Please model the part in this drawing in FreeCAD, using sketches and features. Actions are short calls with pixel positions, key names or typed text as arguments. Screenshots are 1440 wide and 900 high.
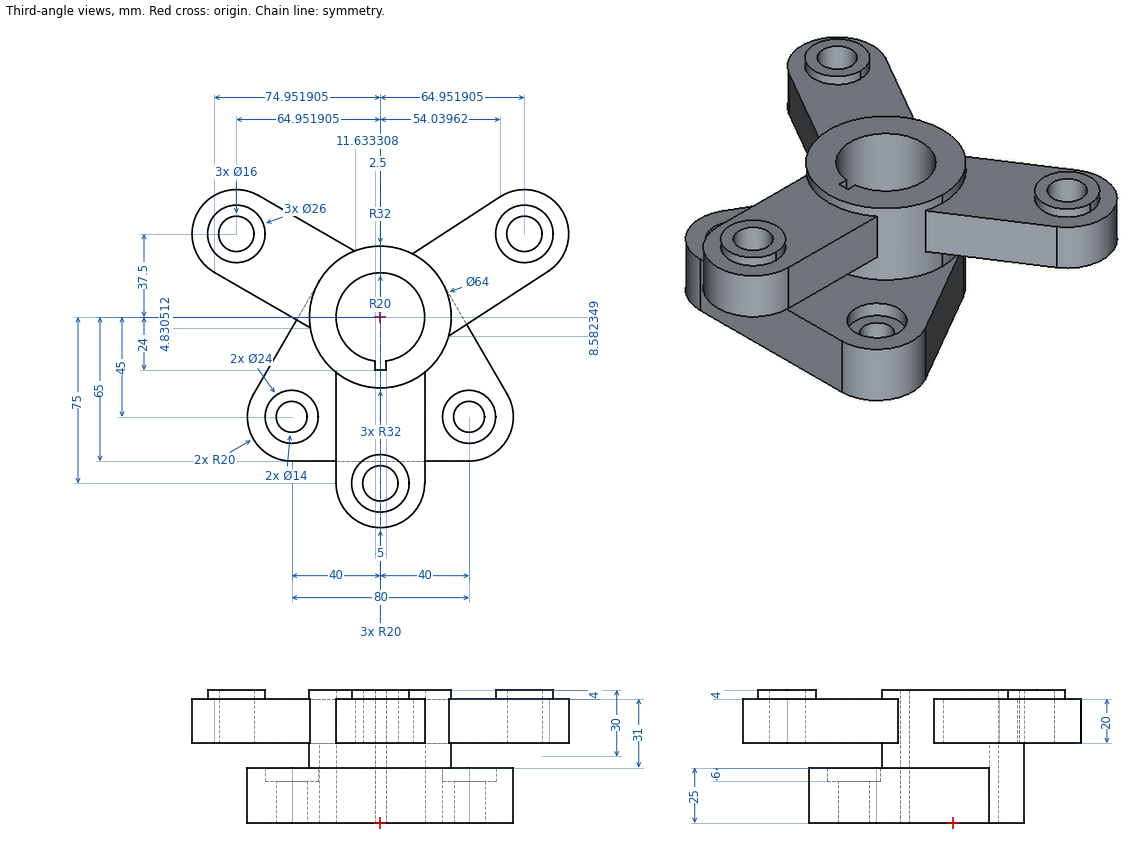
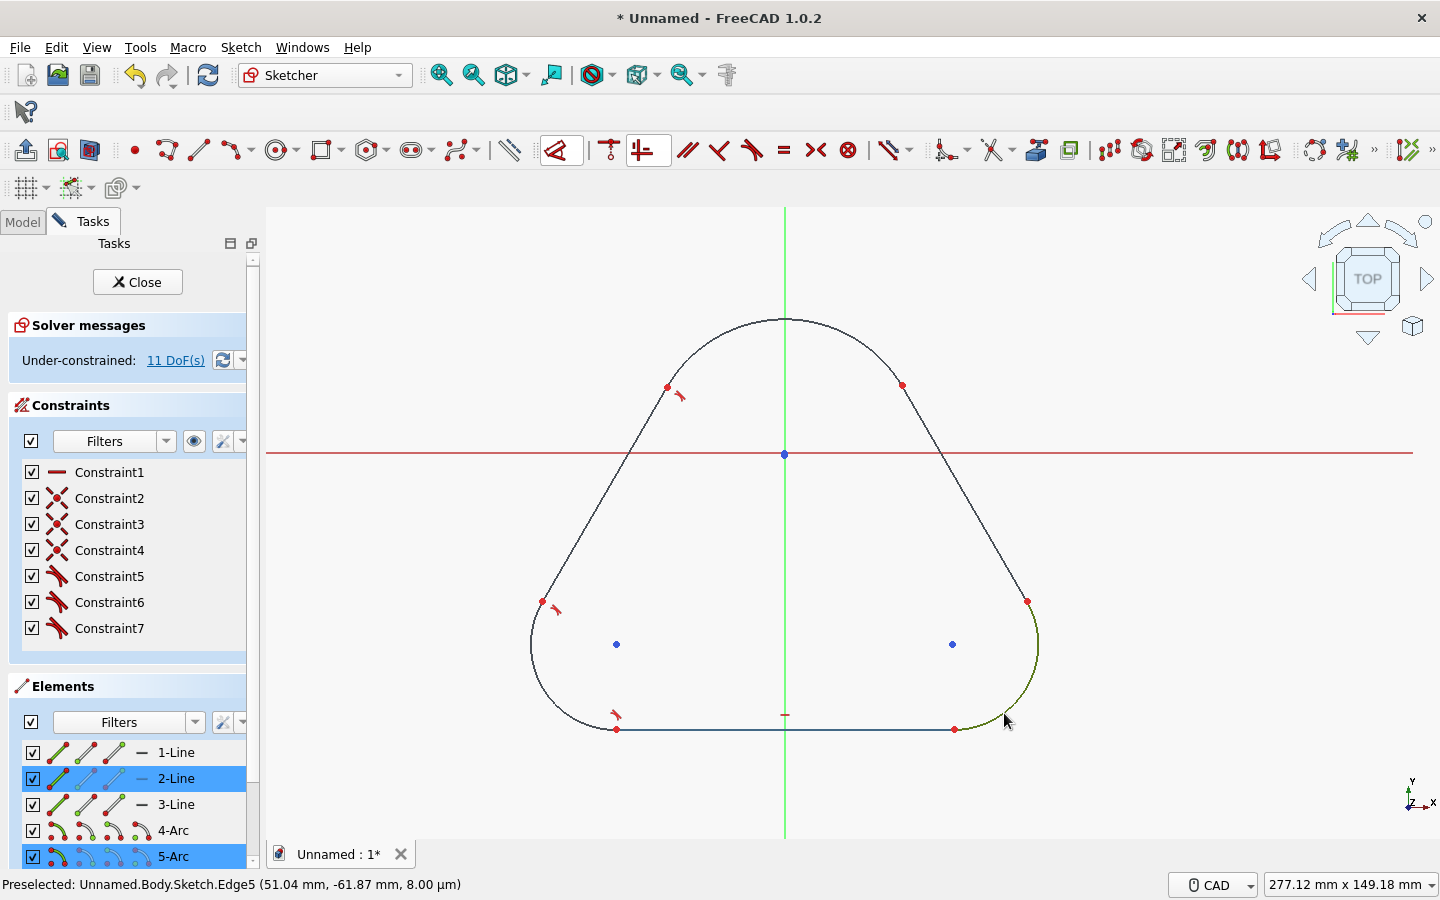
click(752, 150)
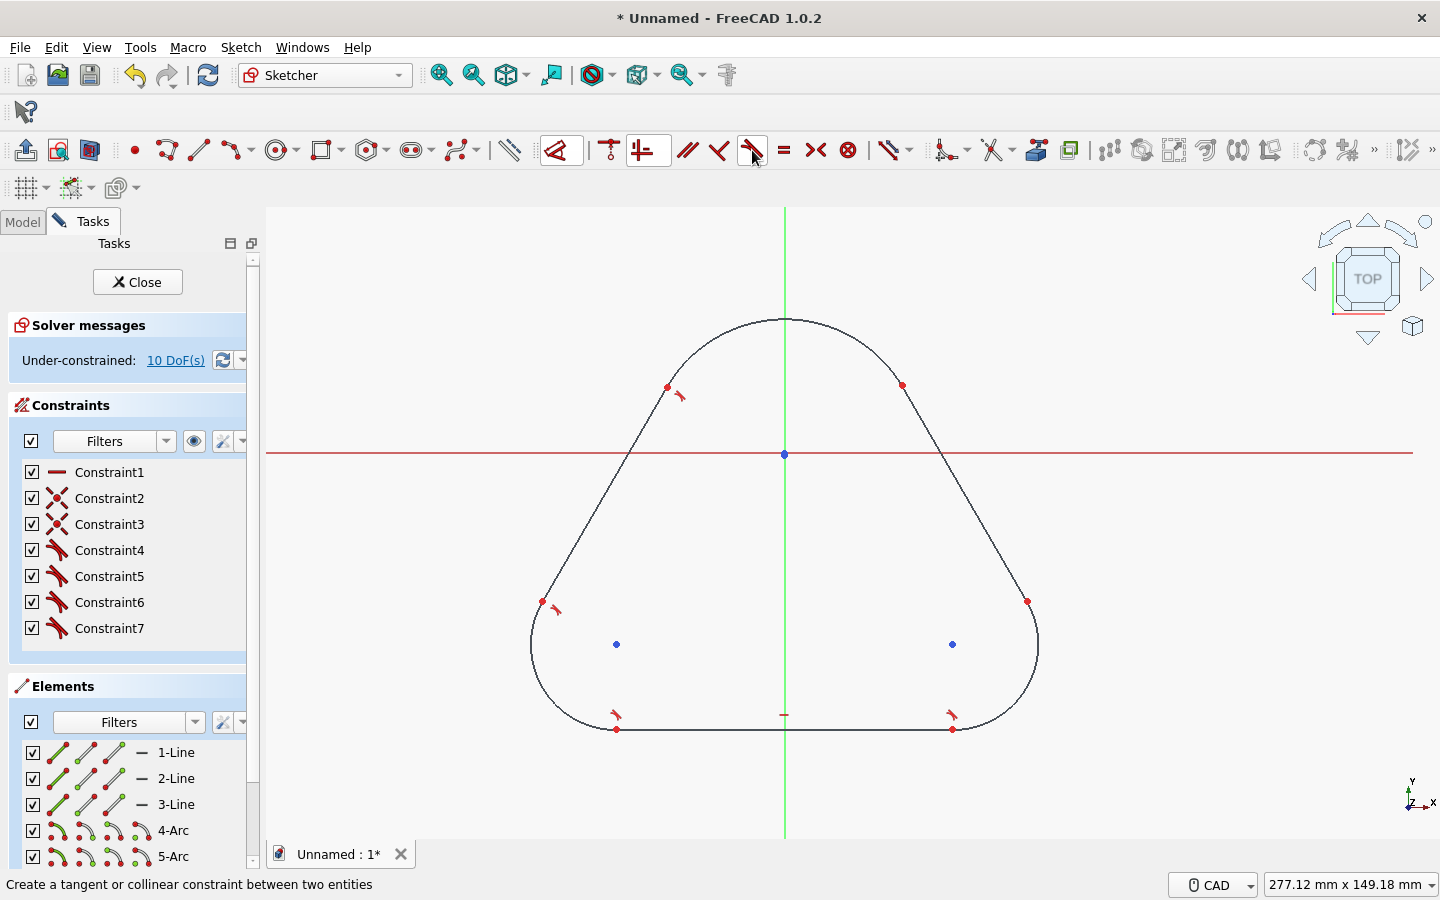
click(990, 537)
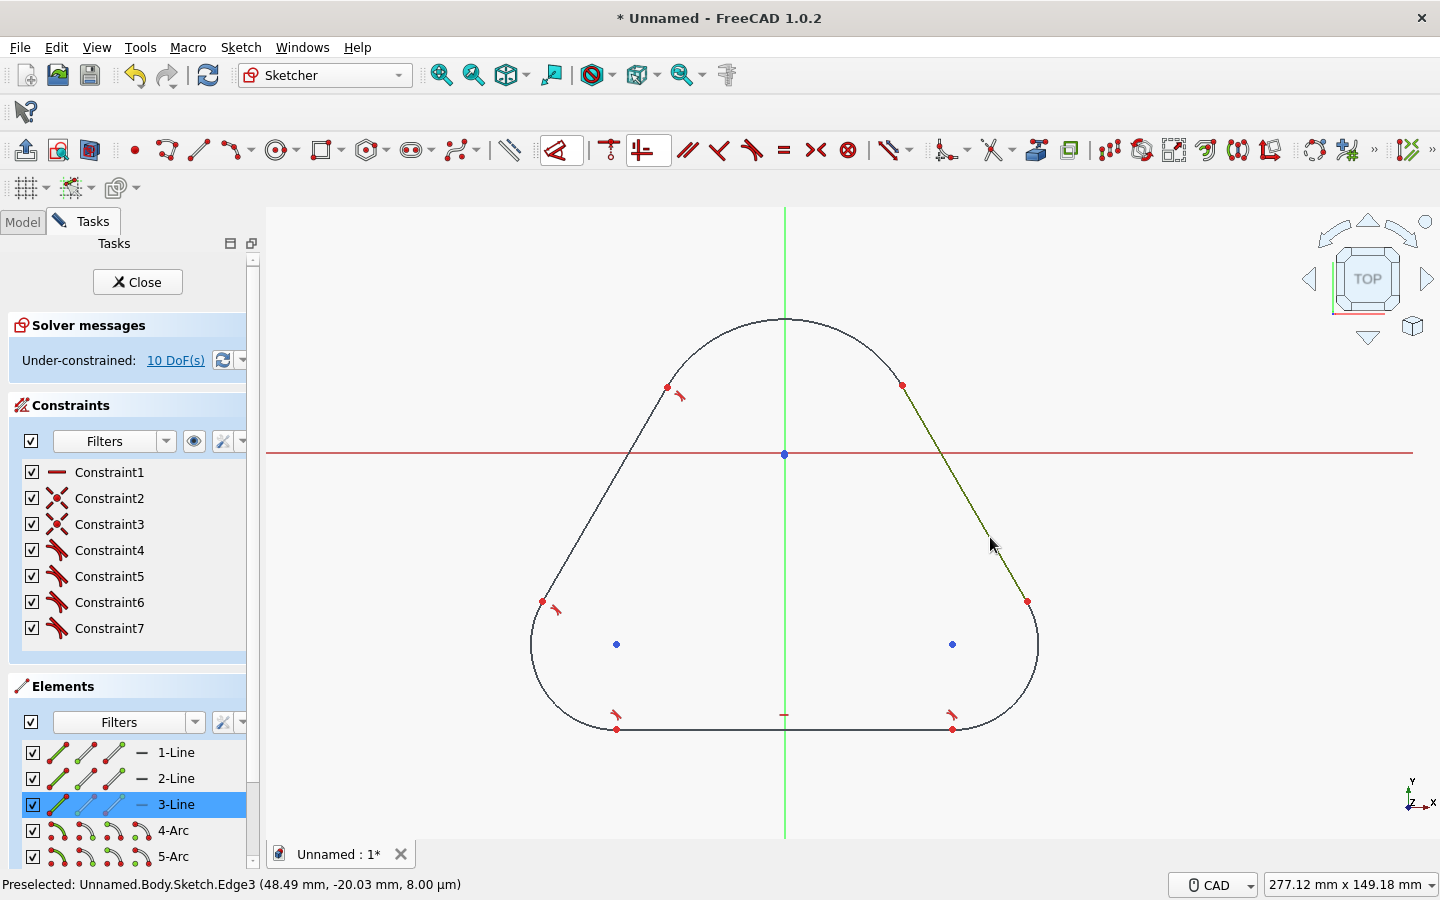
click(1003, 714)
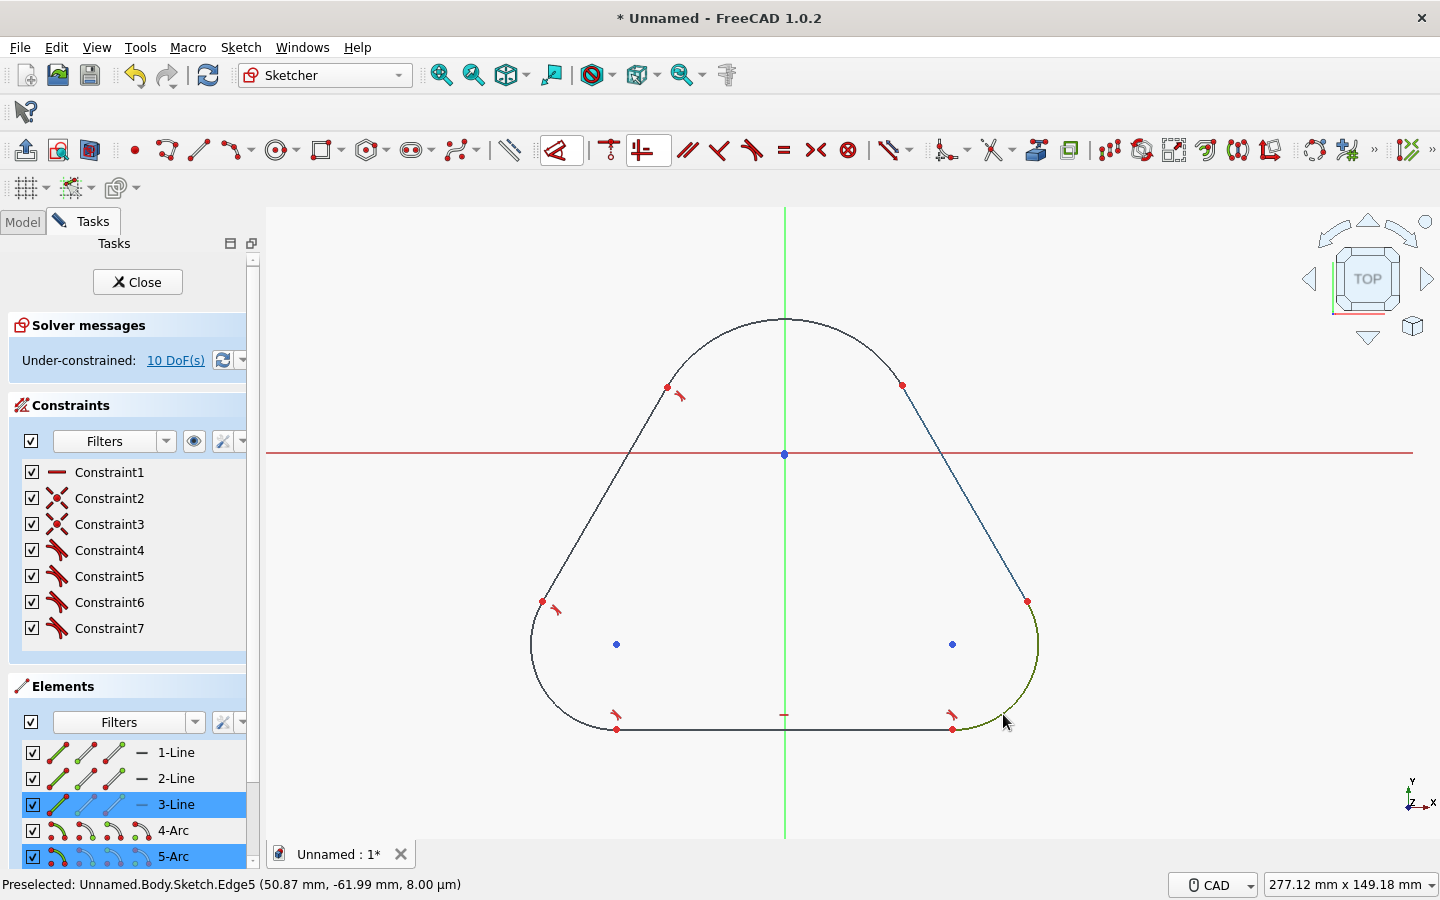
key(t)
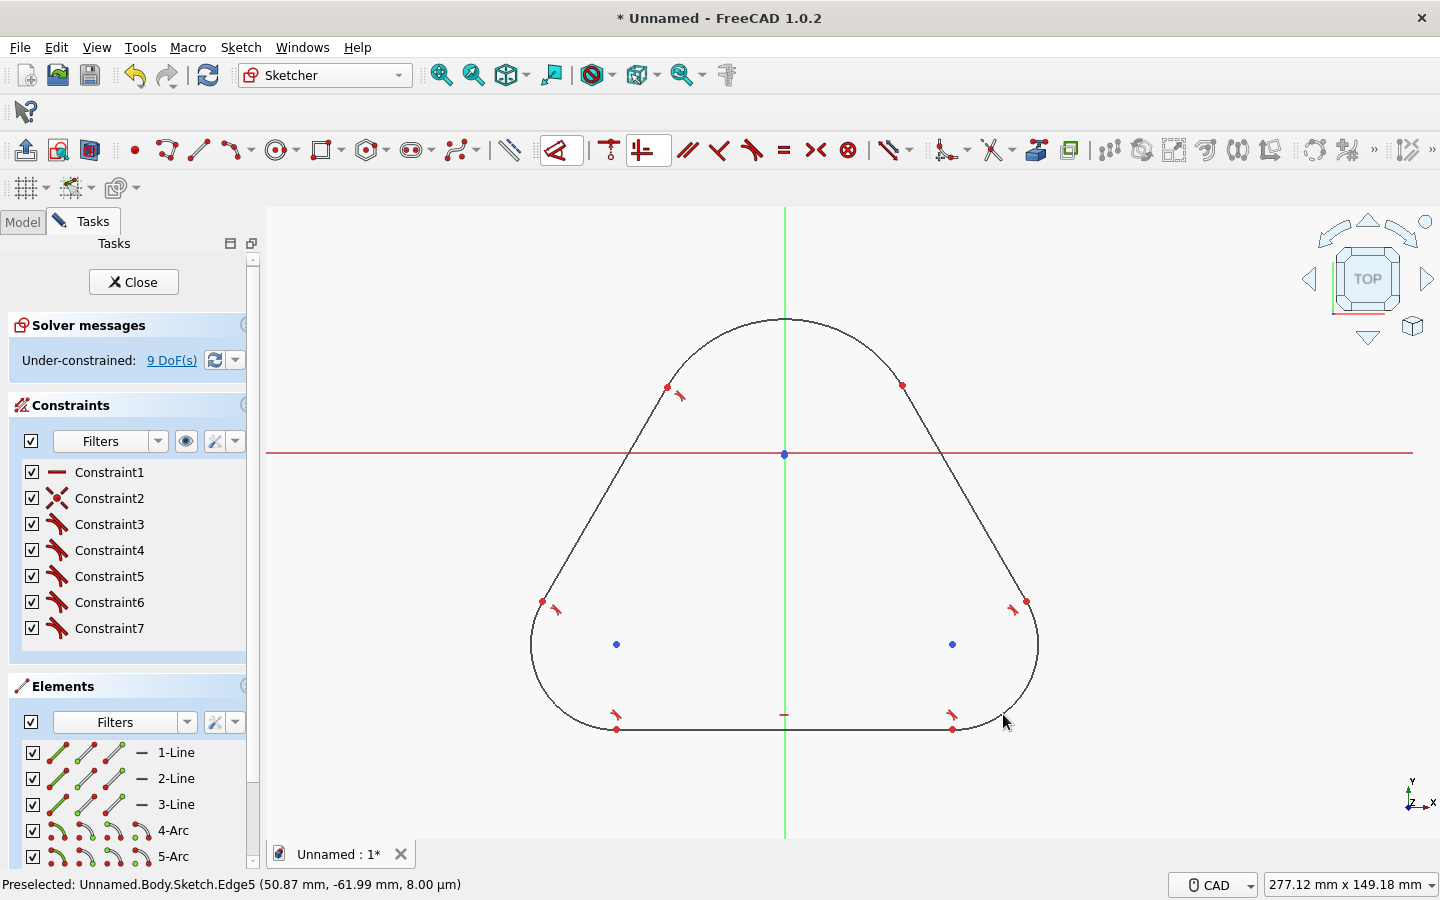
click(989, 537)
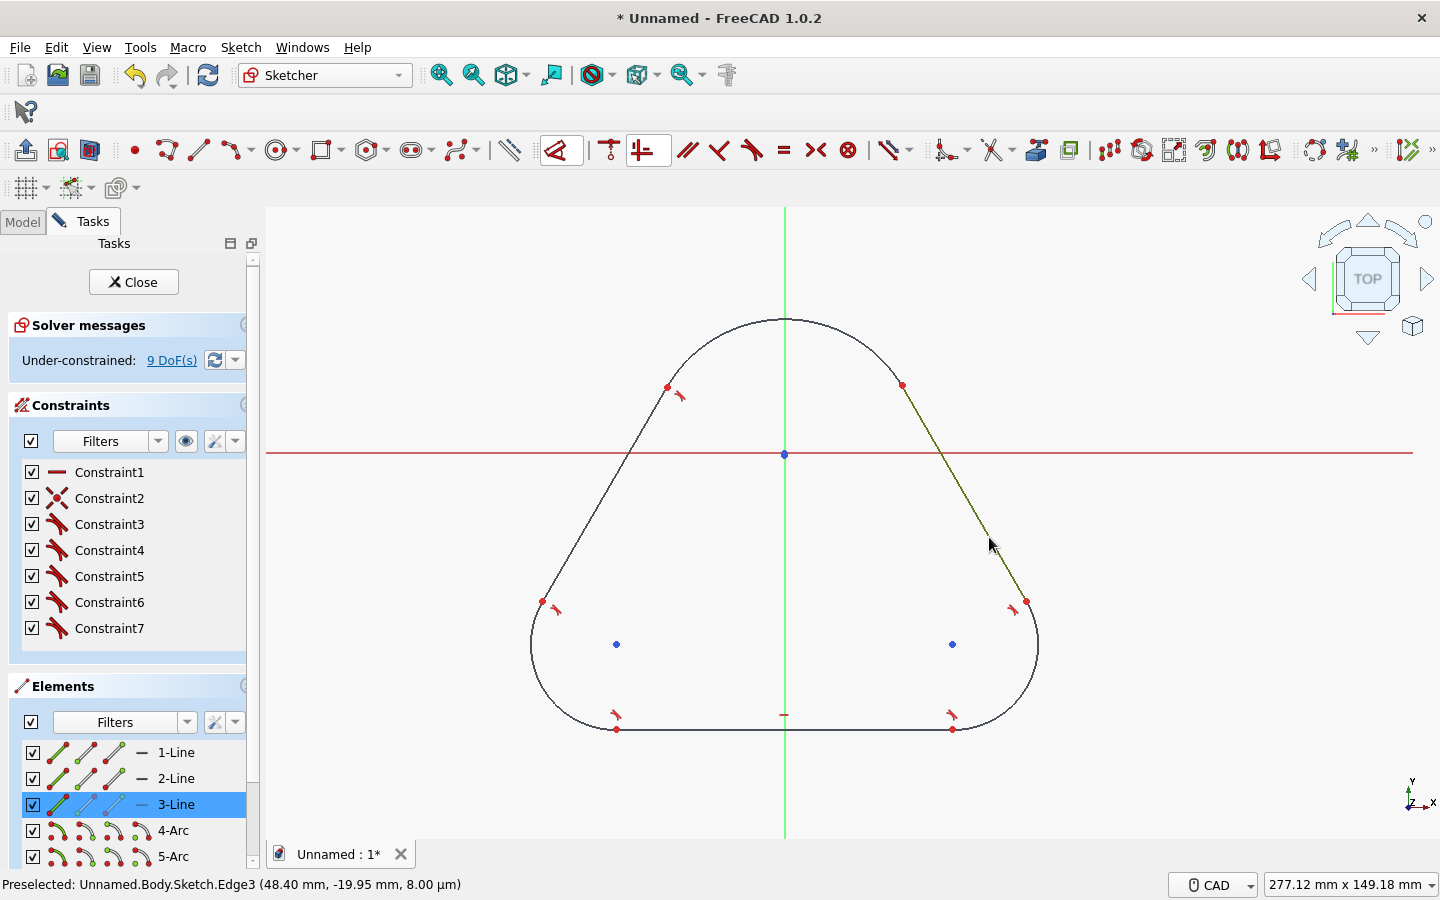
click(839, 331)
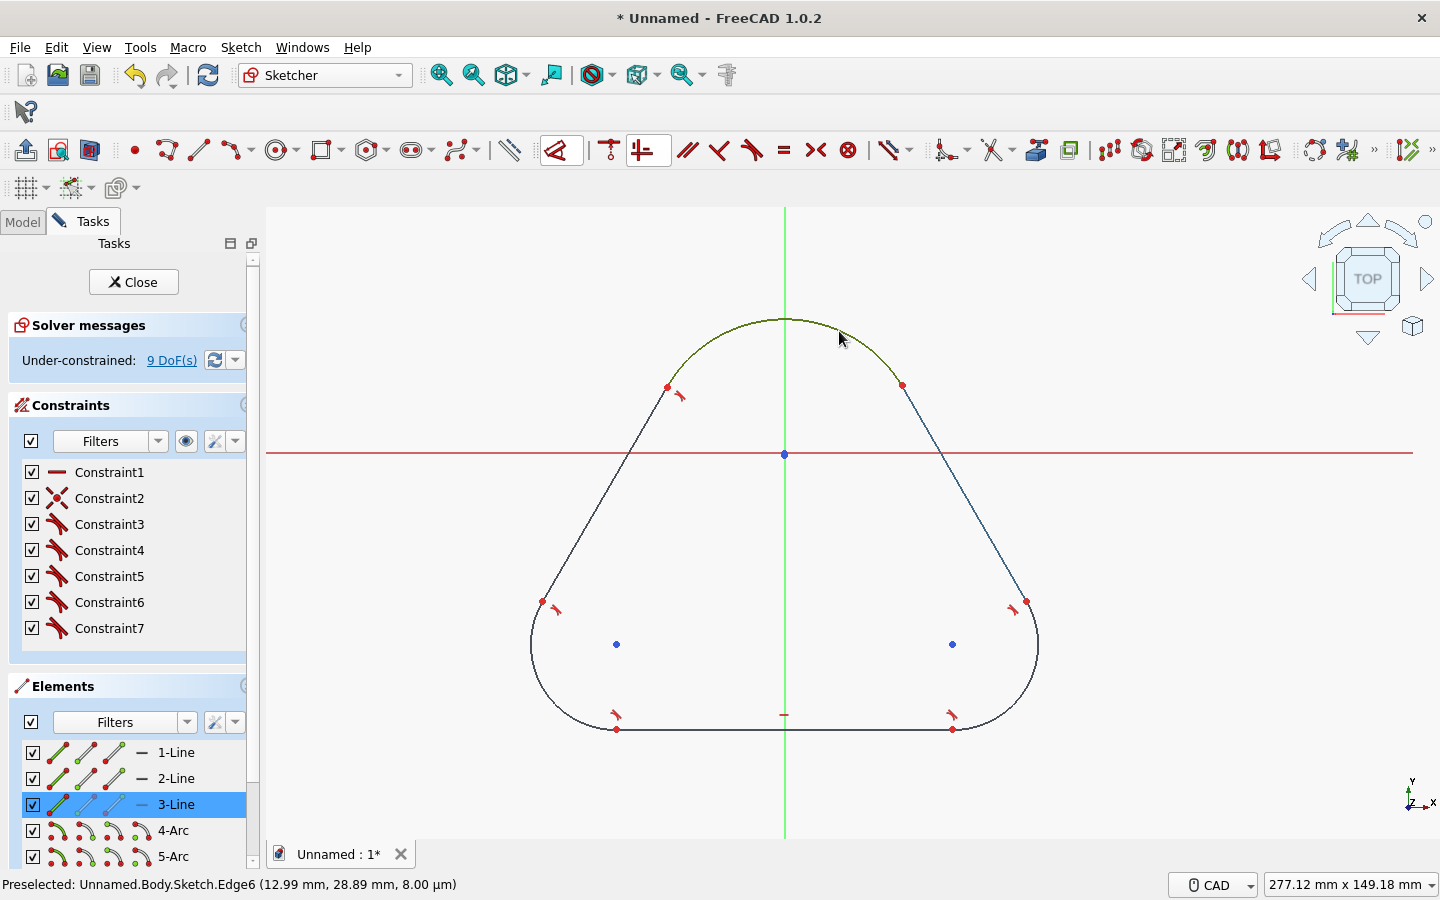
click(752, 150)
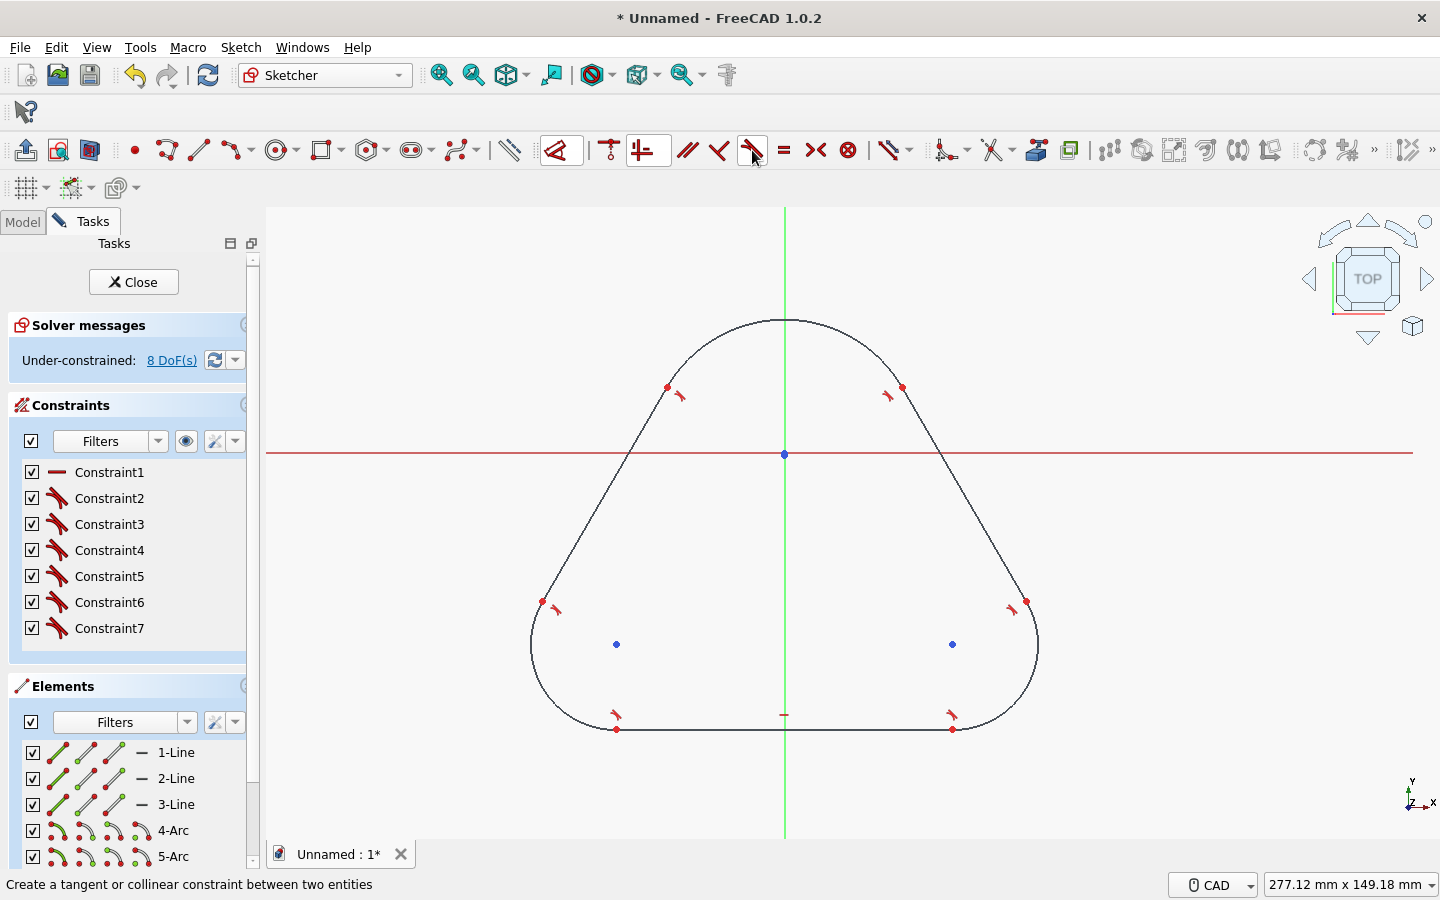
drag(774, 443, 795, 466)